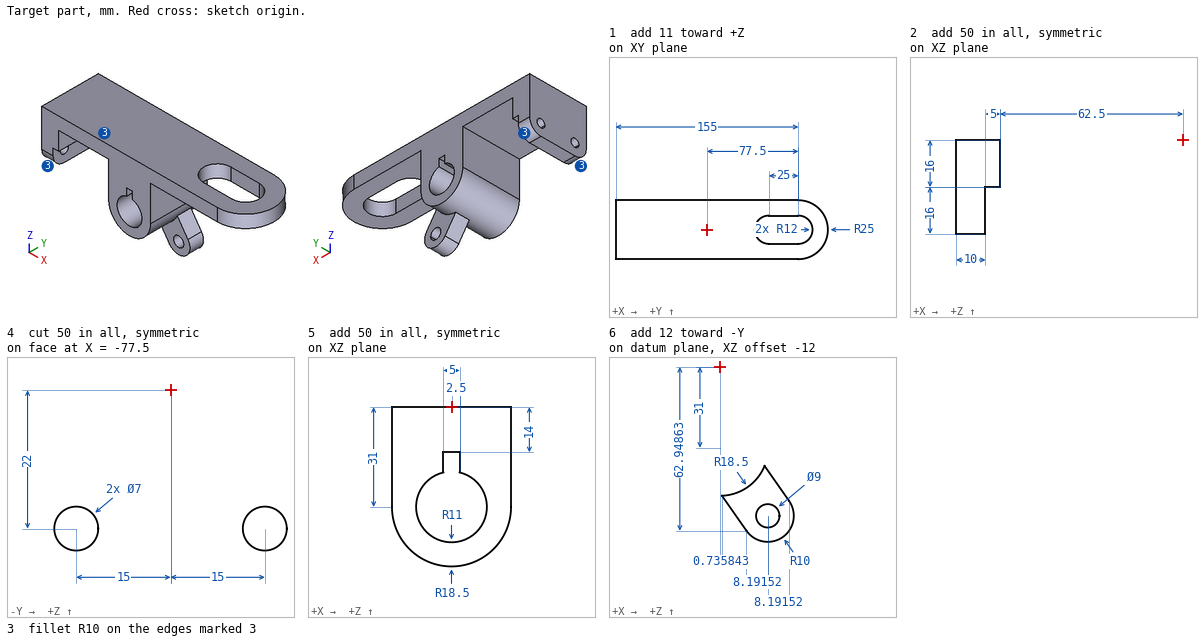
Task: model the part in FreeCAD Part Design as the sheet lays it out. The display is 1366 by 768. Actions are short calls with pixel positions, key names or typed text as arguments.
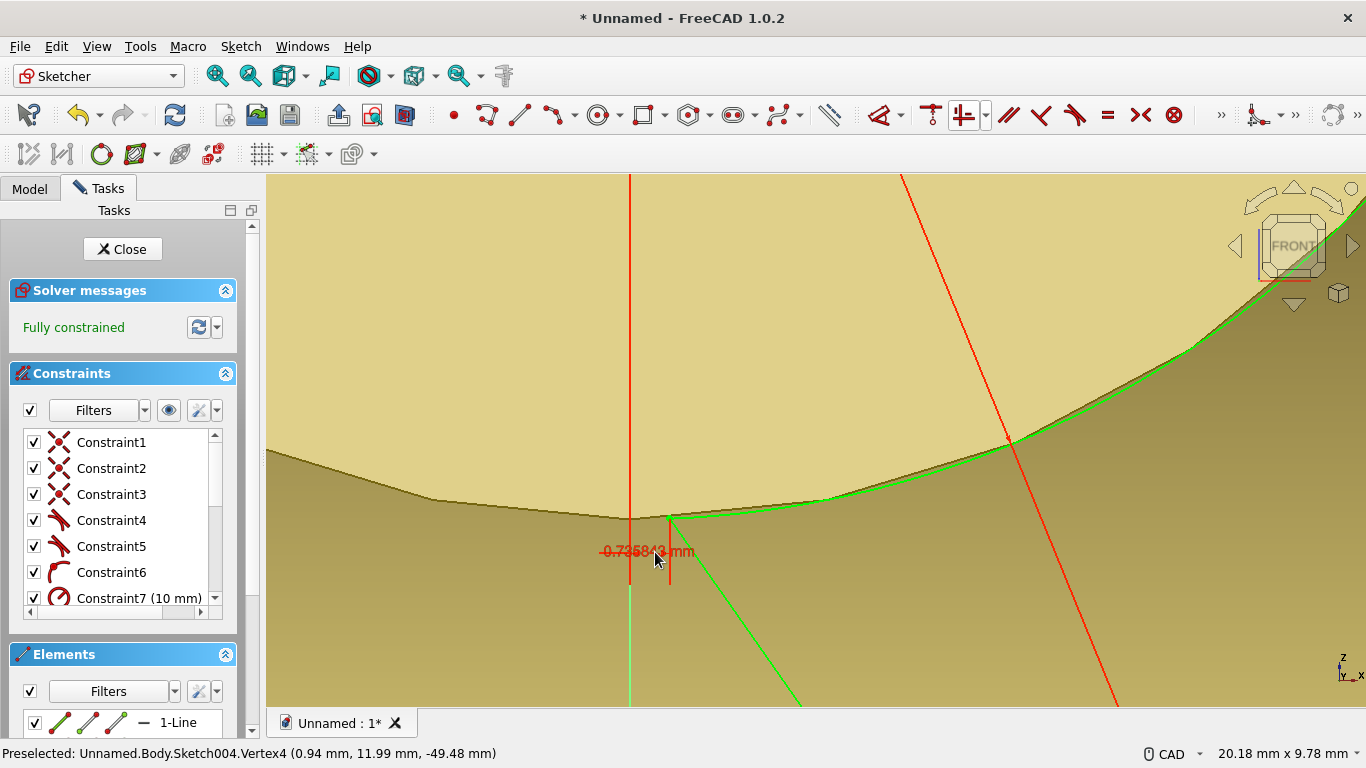
click(123, 249)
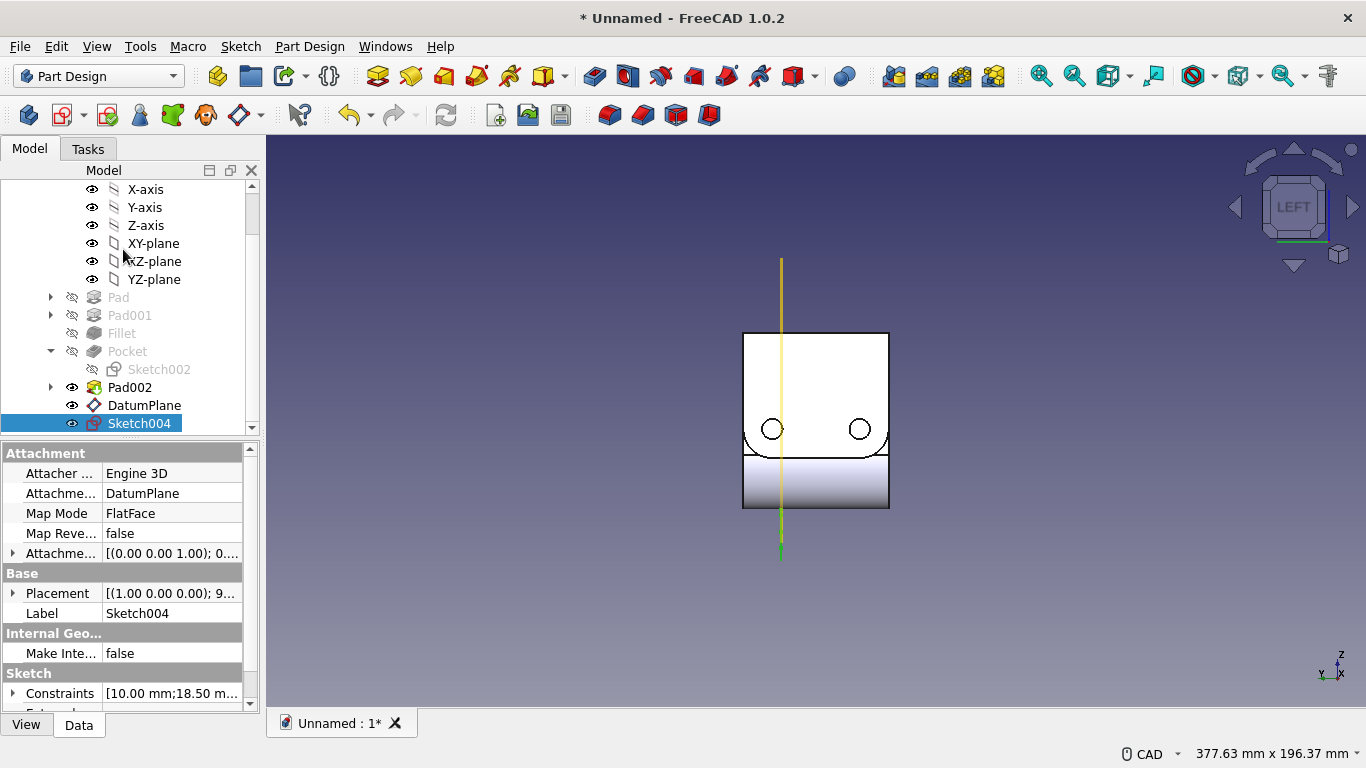
click(378, 76)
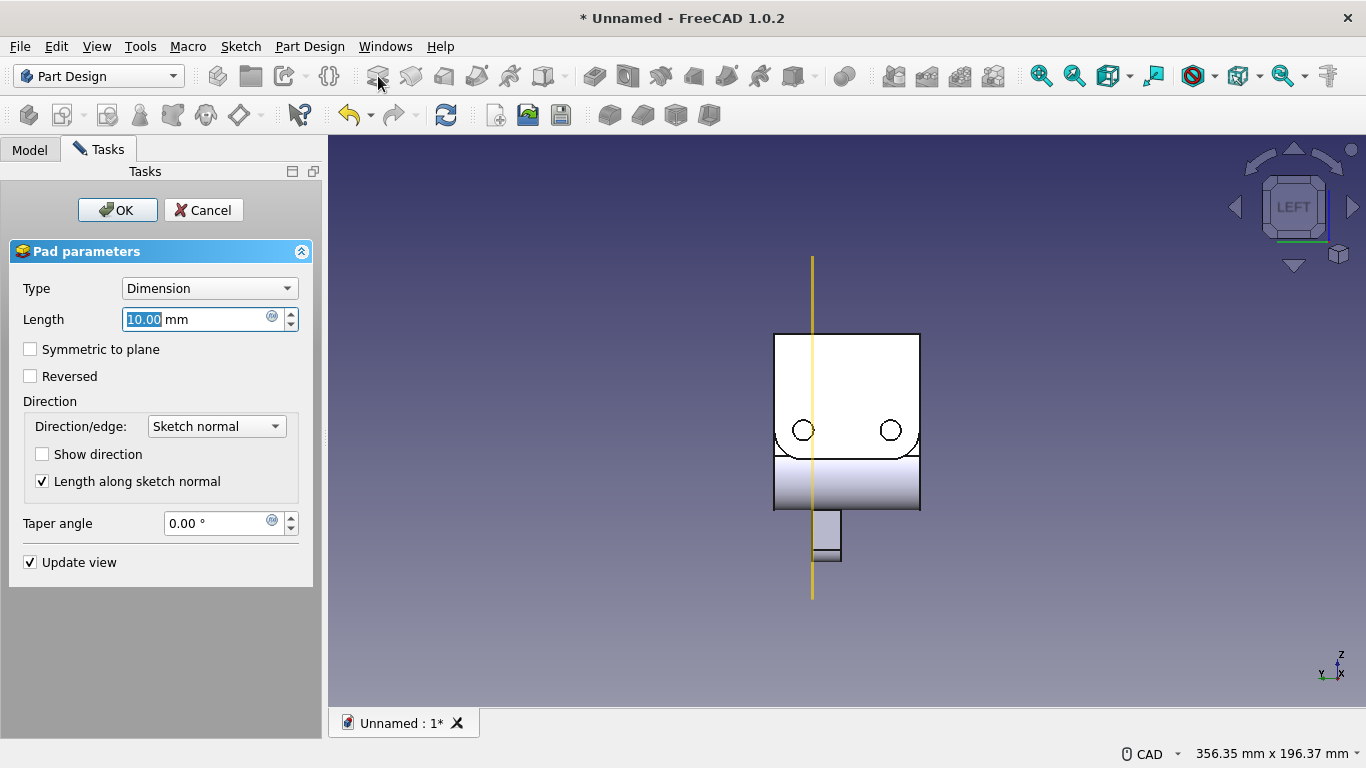
text(12)
key(Tab)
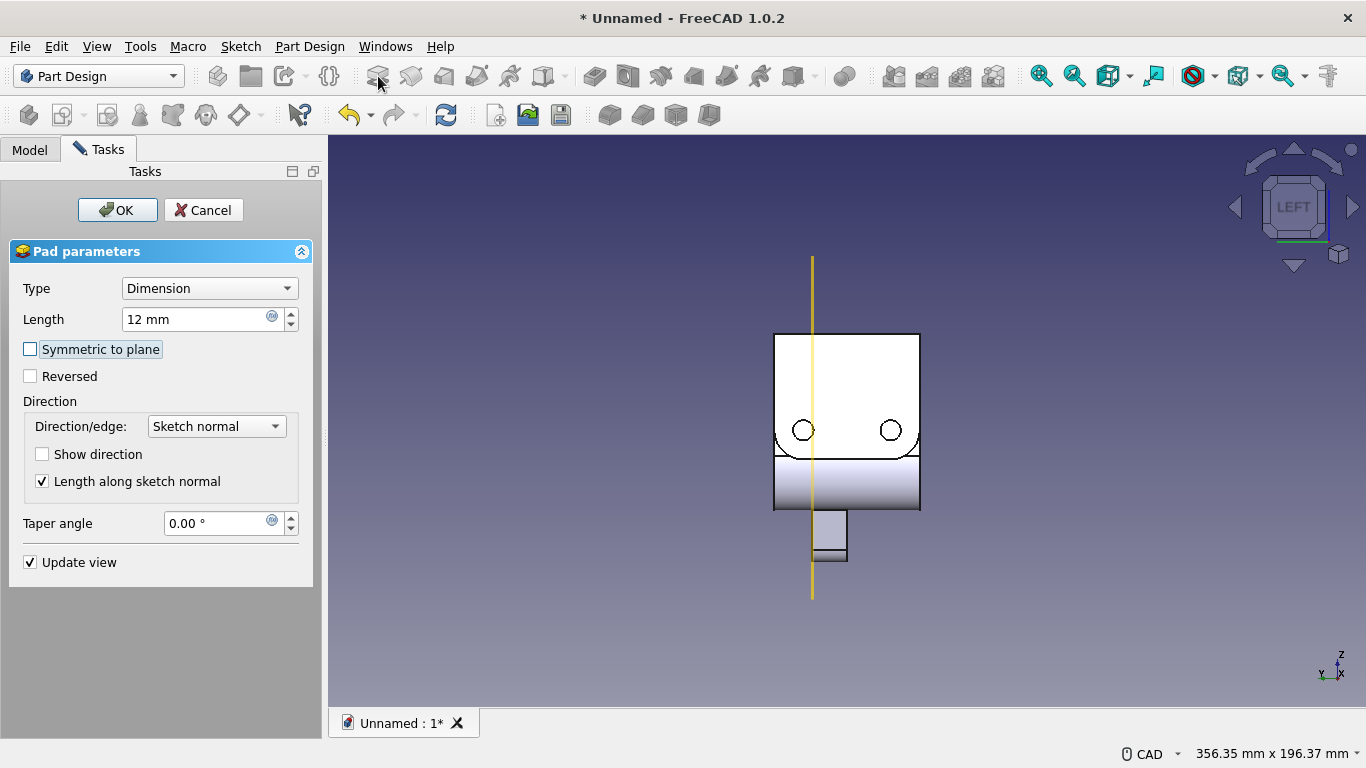
click(118, 210)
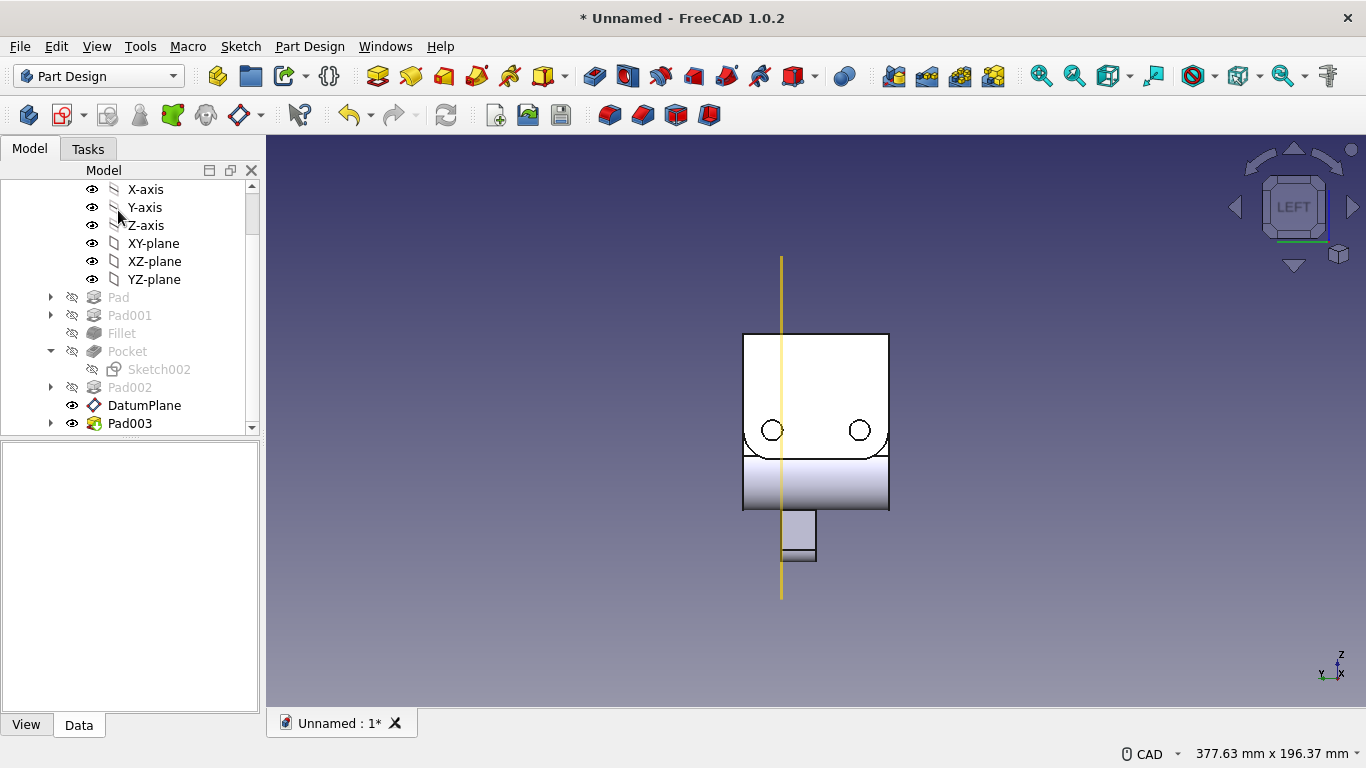
click(117, 405)
key(space)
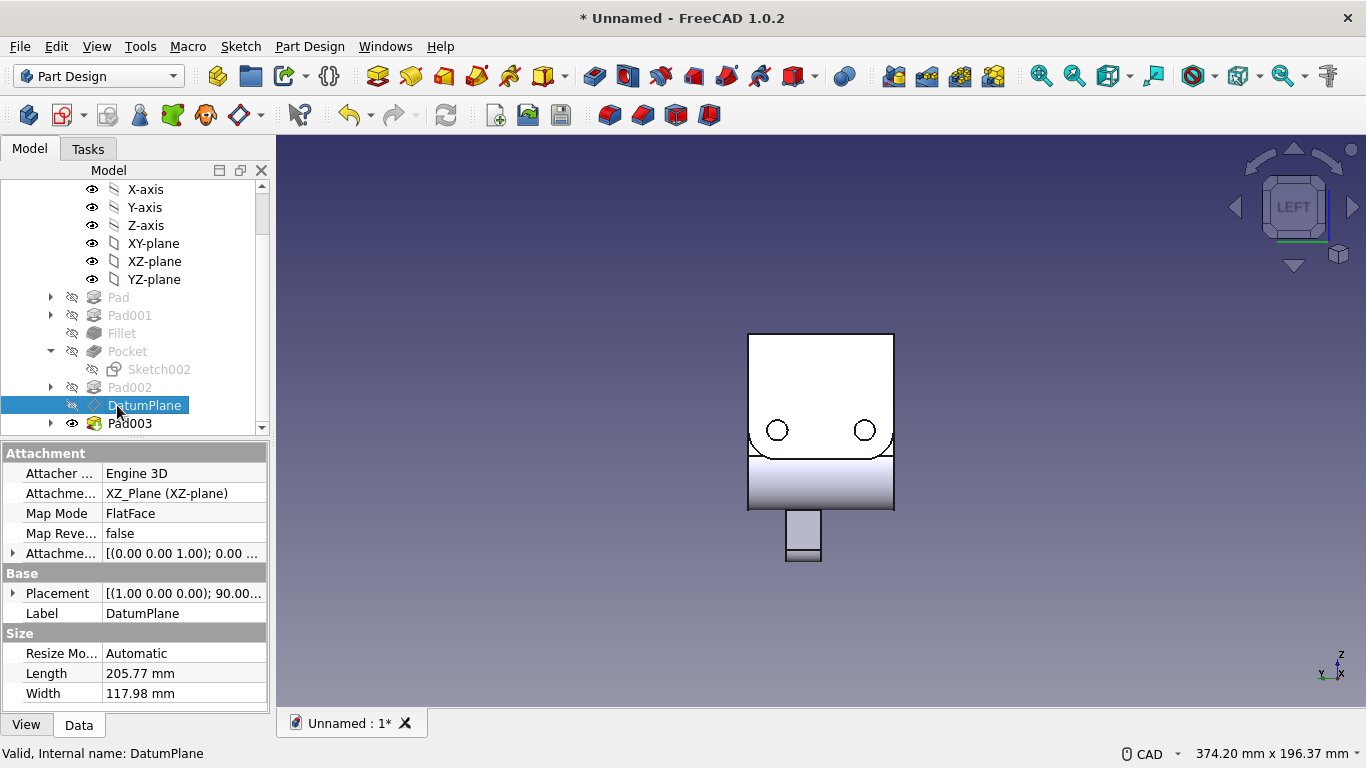
key(0)